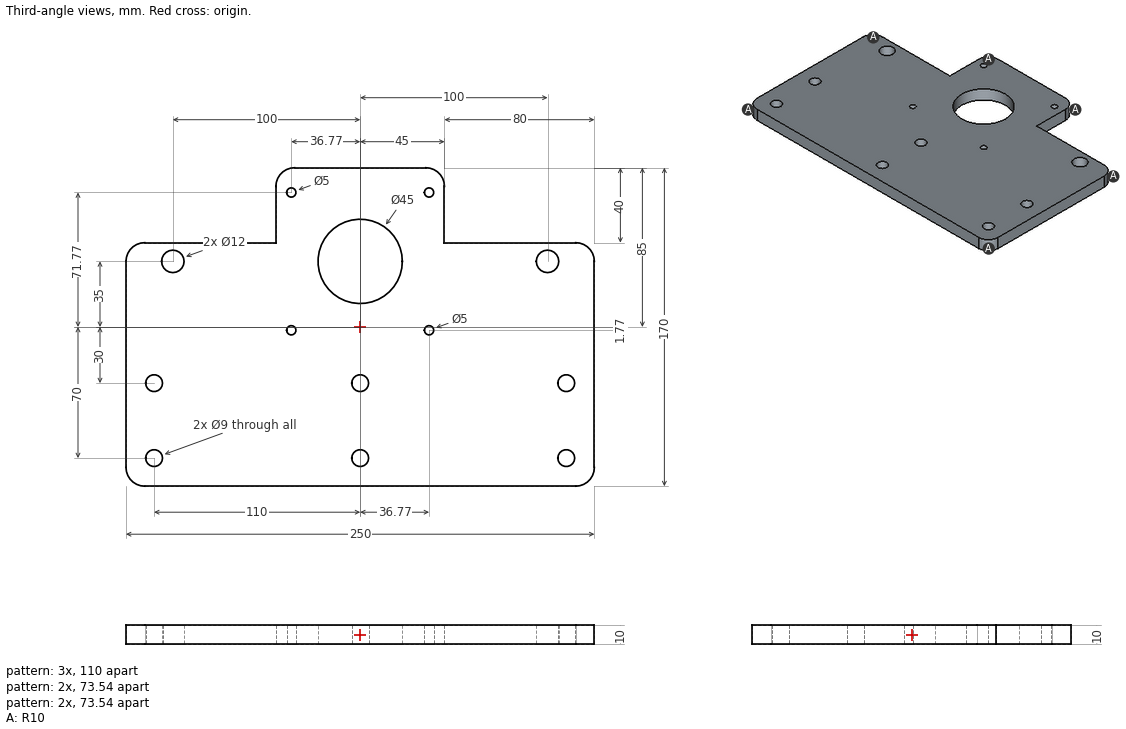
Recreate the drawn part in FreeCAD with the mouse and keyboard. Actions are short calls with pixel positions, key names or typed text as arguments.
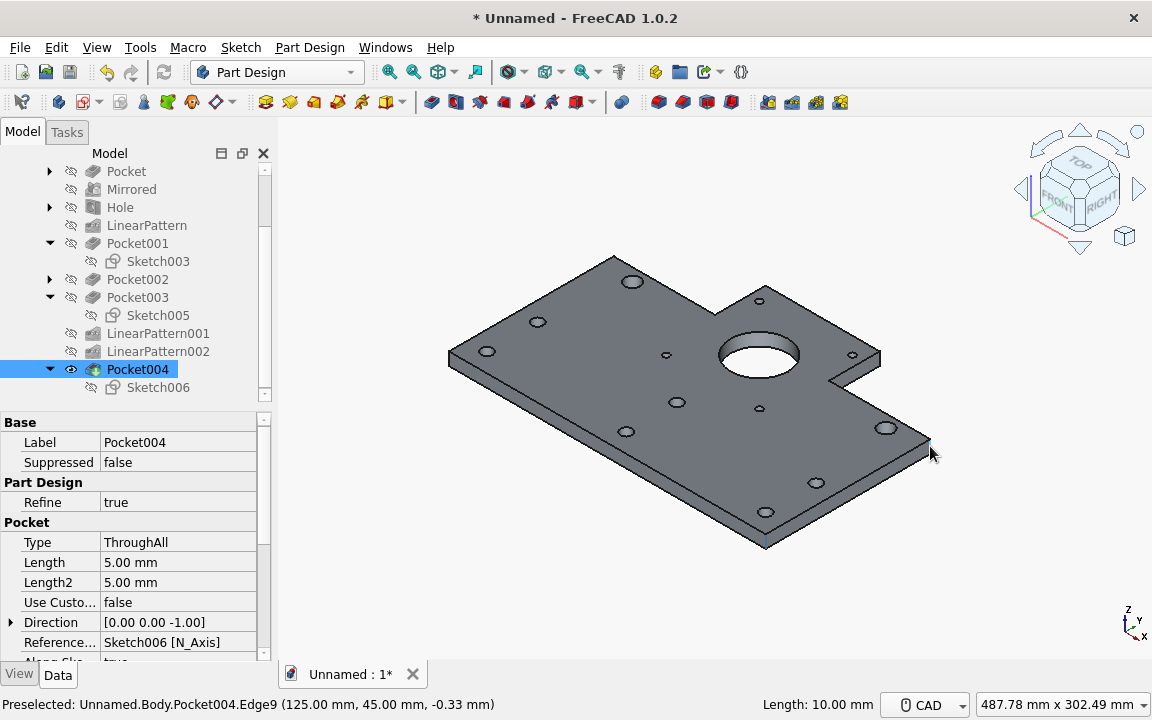
key(2)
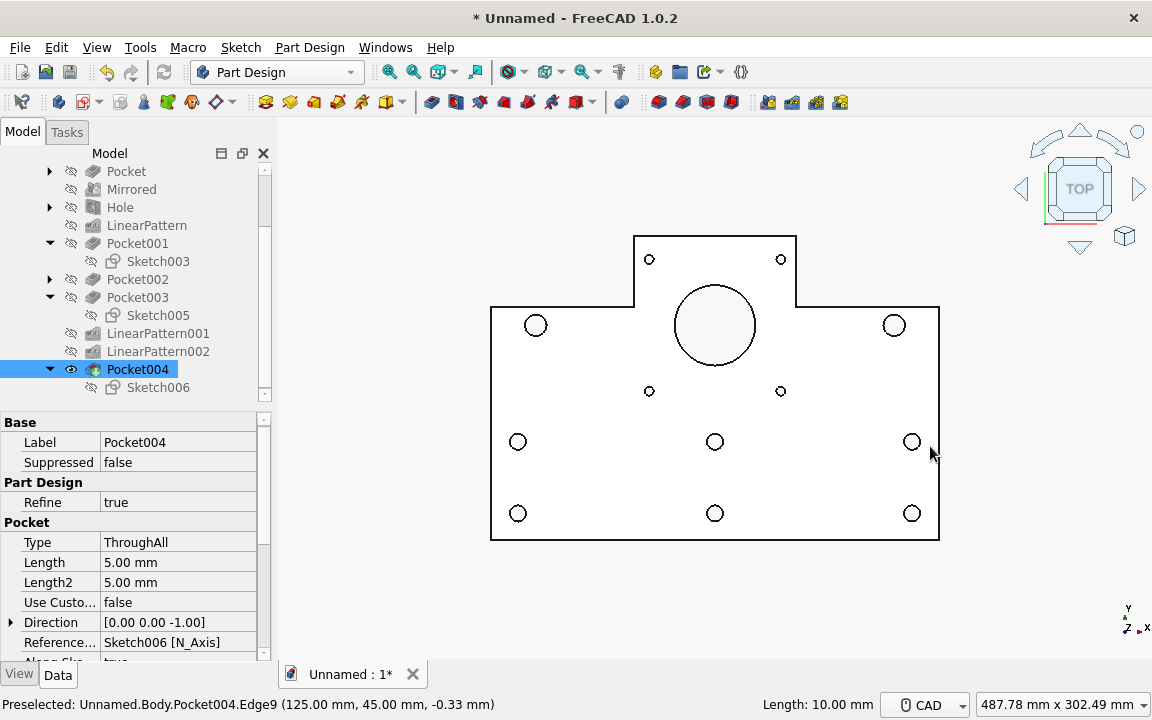
scroll(939, 306, up, 5)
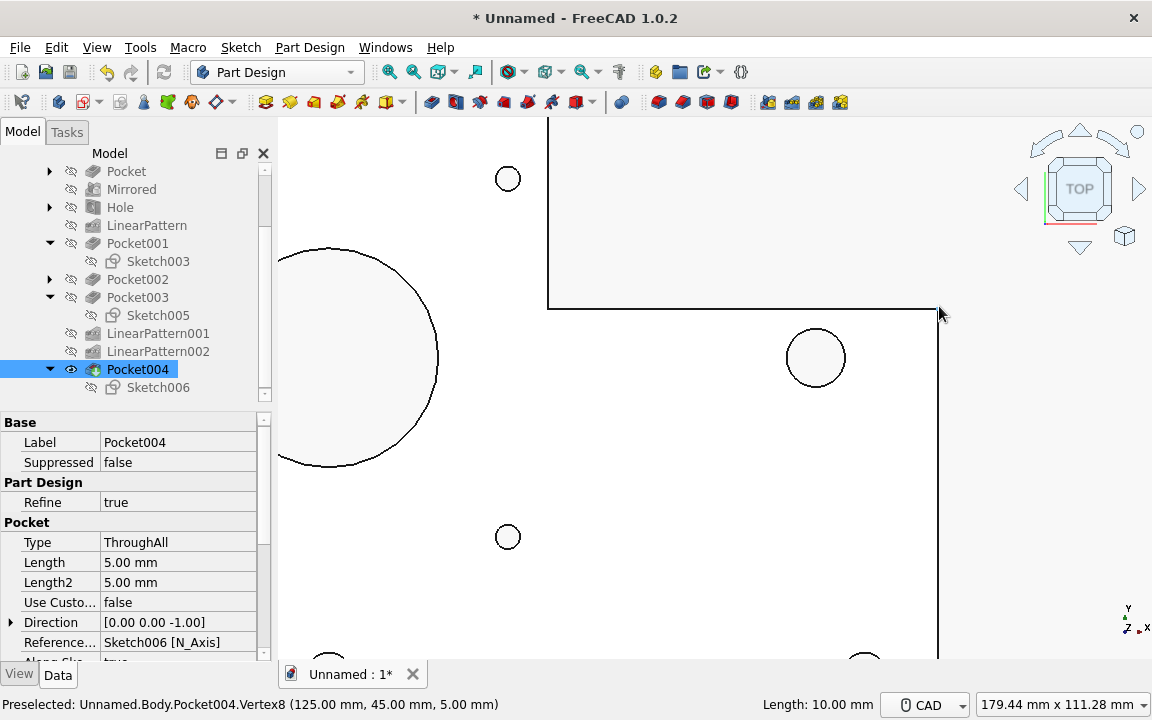
click(390, 72)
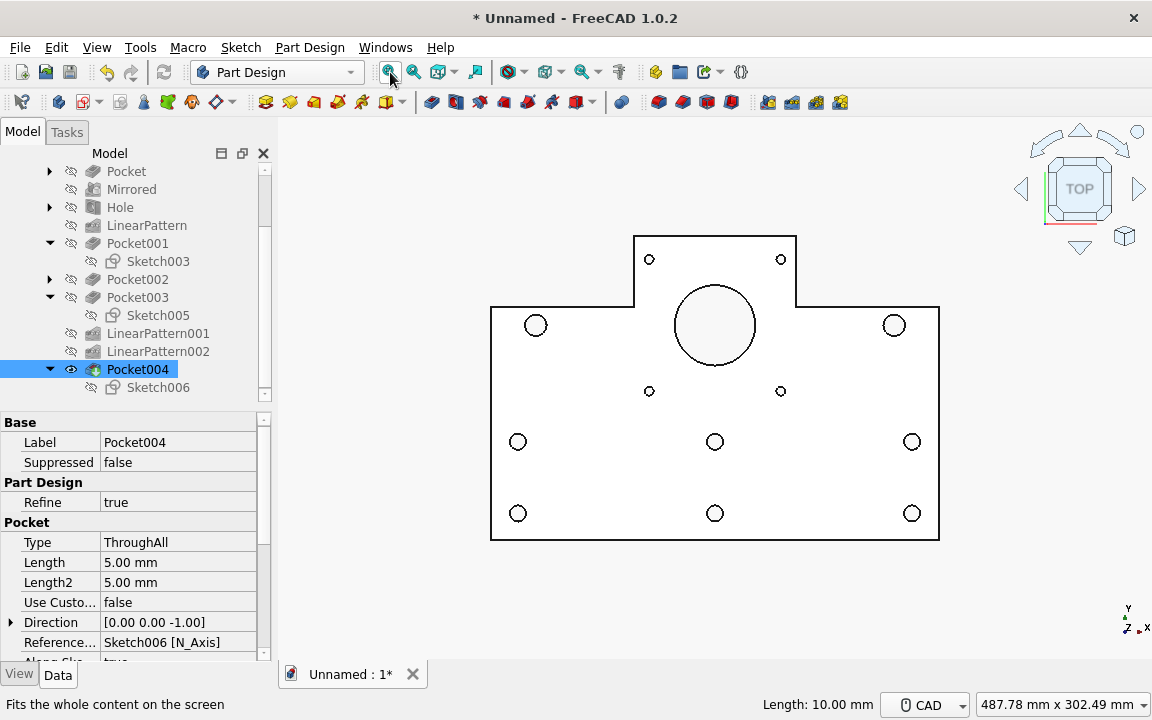
key(1)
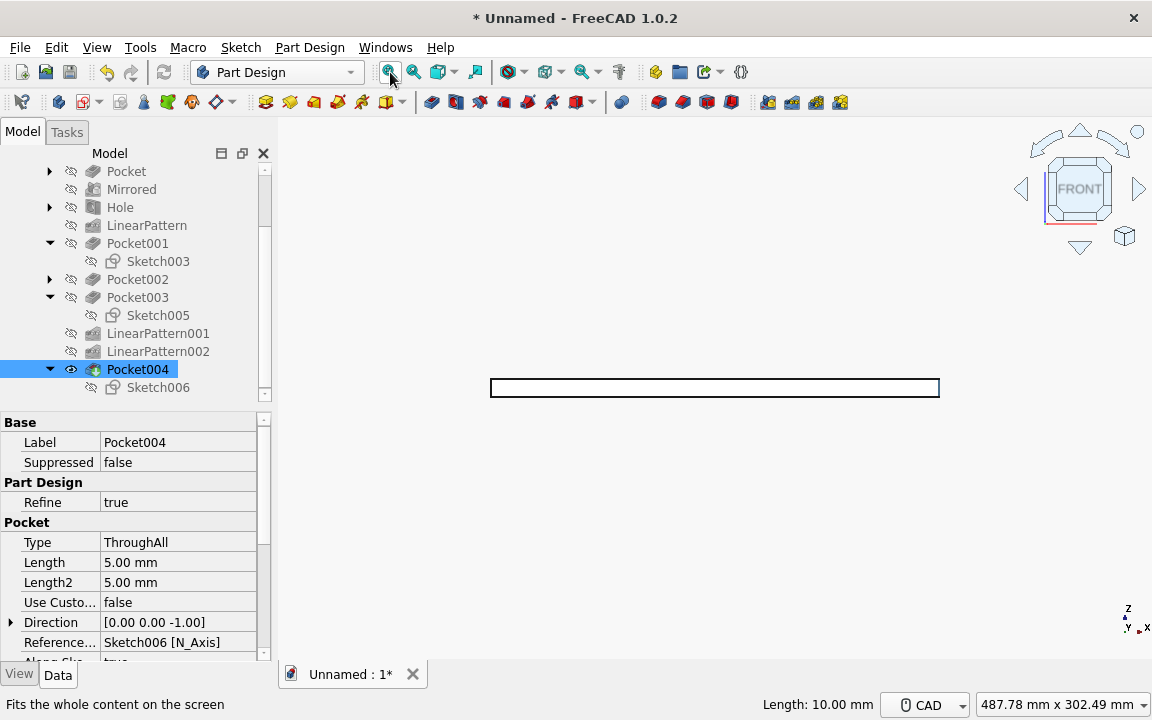
click(491, 387, ctrl)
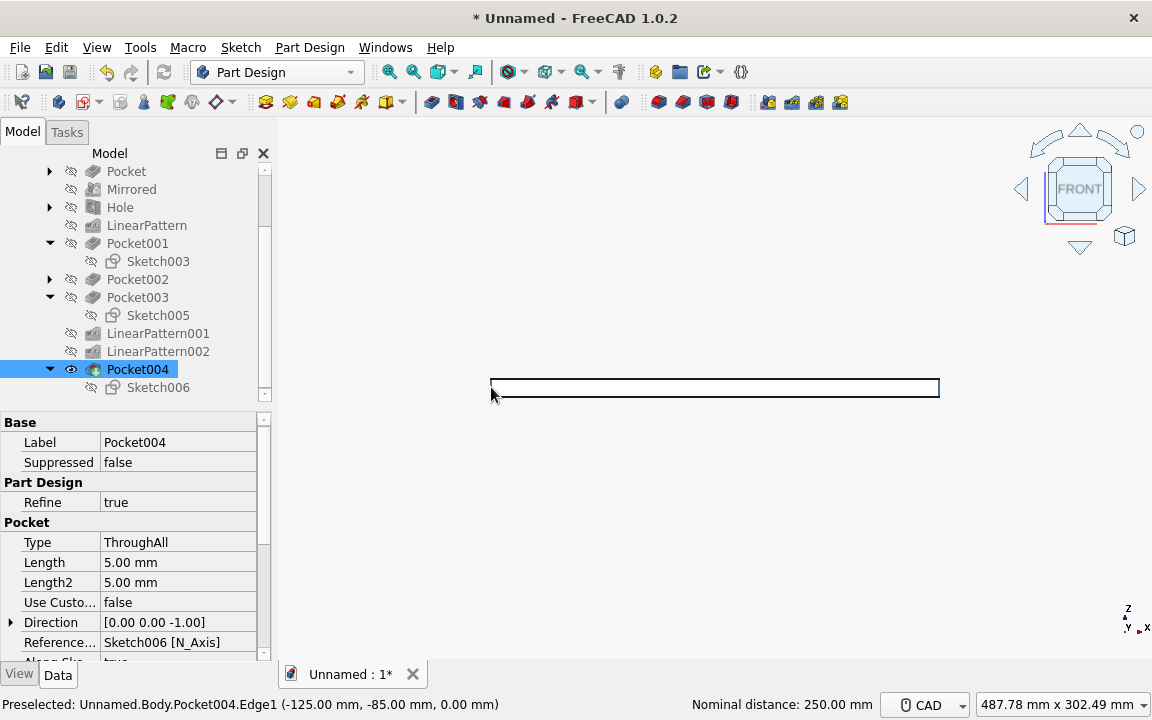
scroll(939, 387, up, 5)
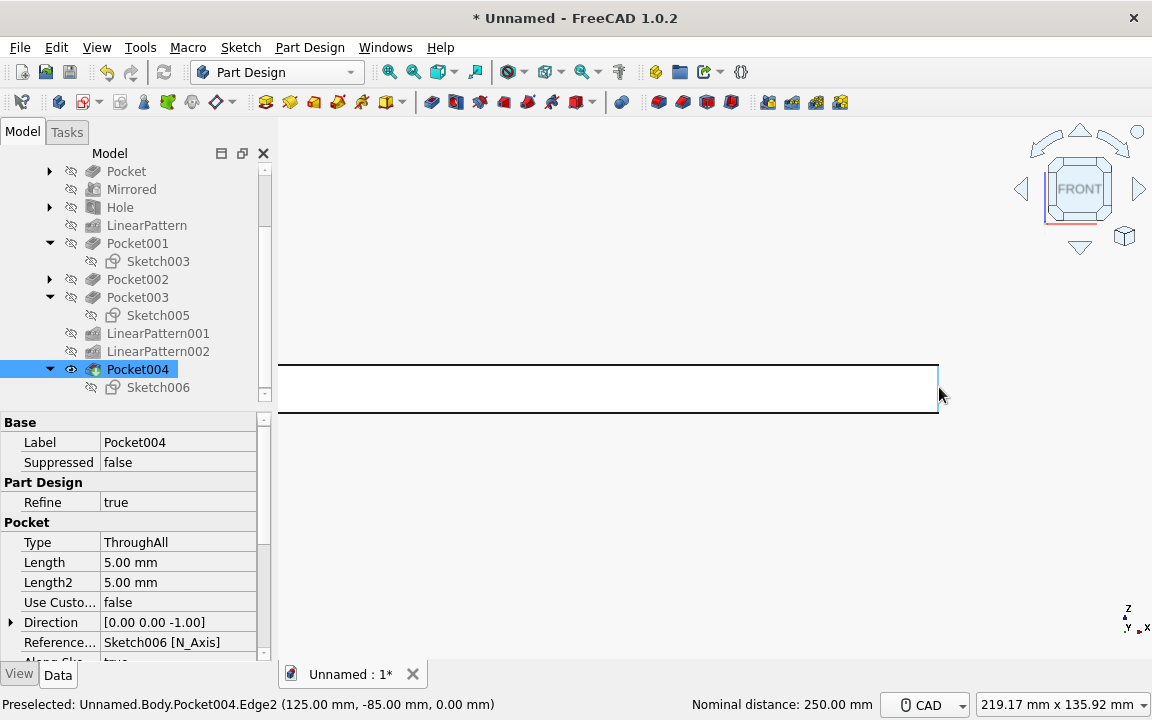
key(v)
key(f)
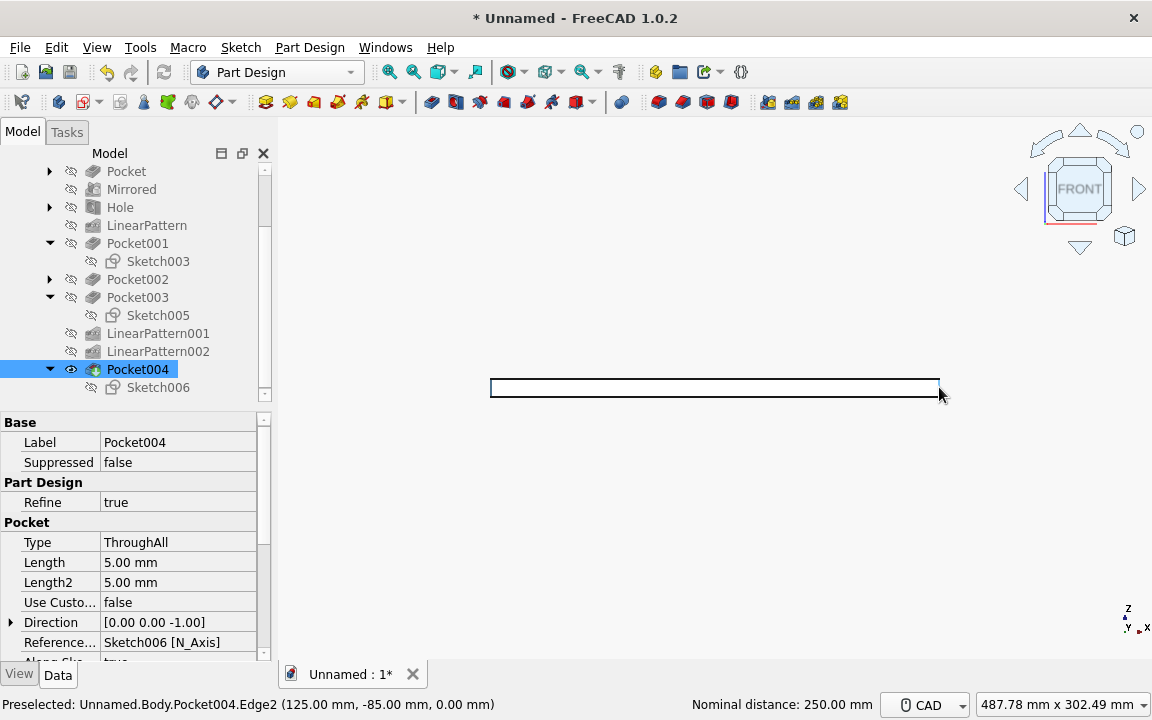
key(3)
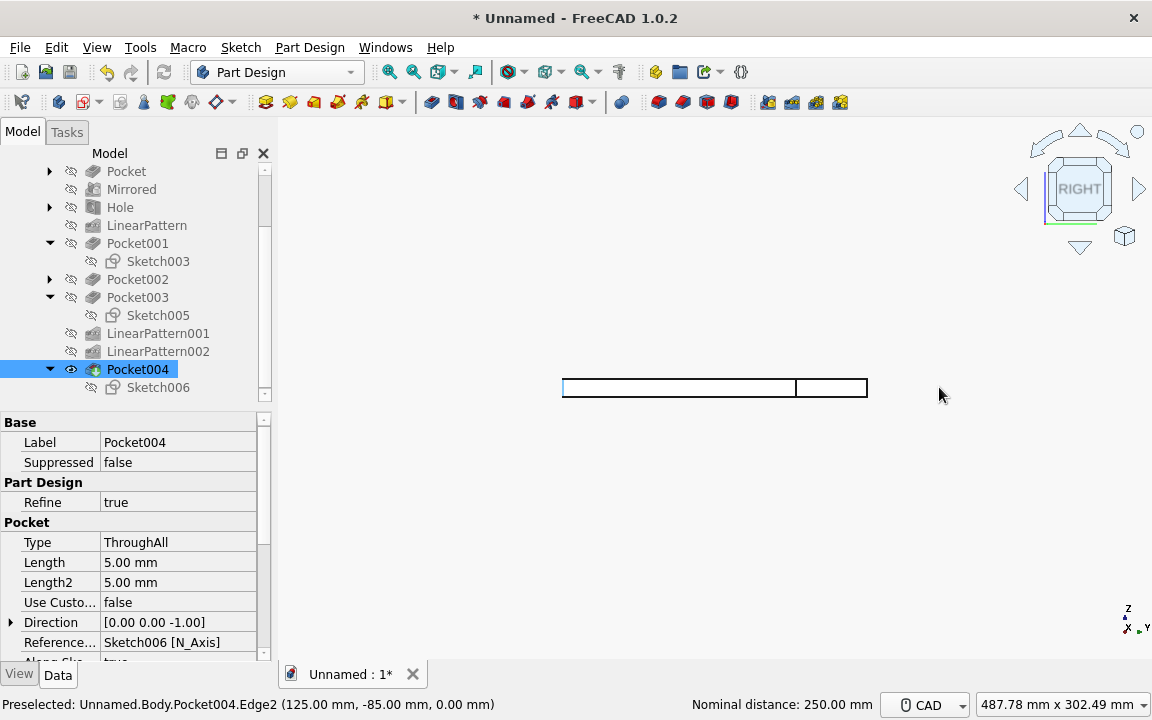
key(v)
key(f)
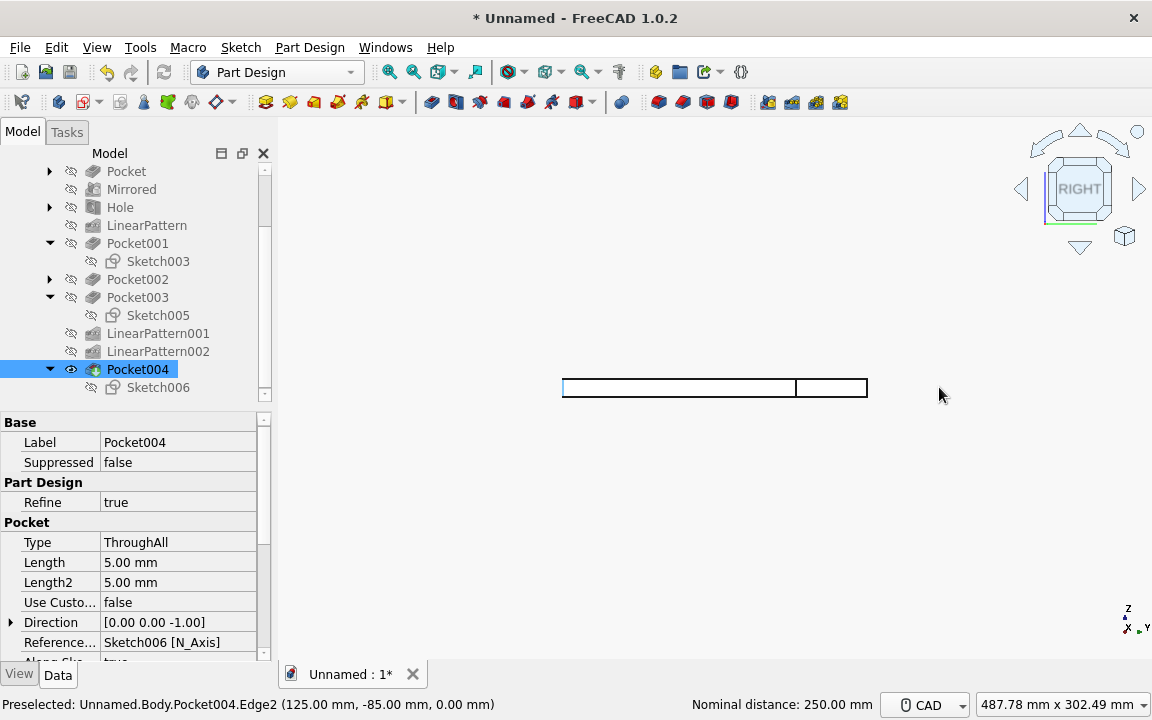
click(796, 387, ctrl)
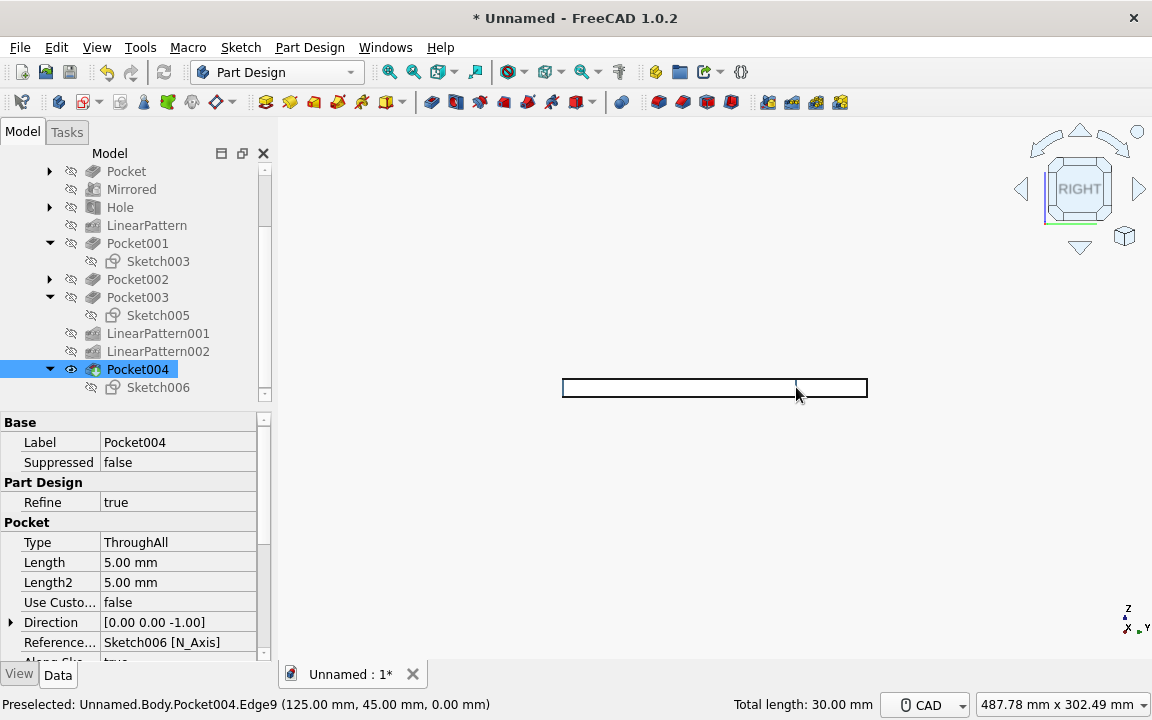
click(867, 387, ctrl)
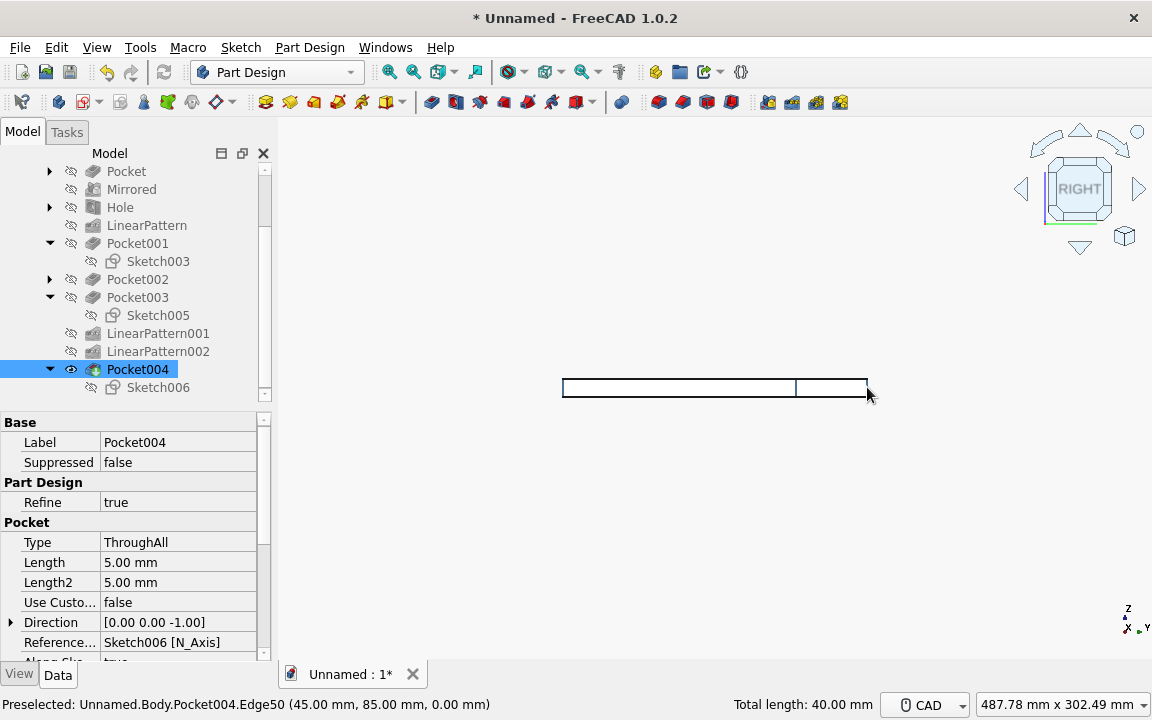
scroll(796, 387, up, 5)